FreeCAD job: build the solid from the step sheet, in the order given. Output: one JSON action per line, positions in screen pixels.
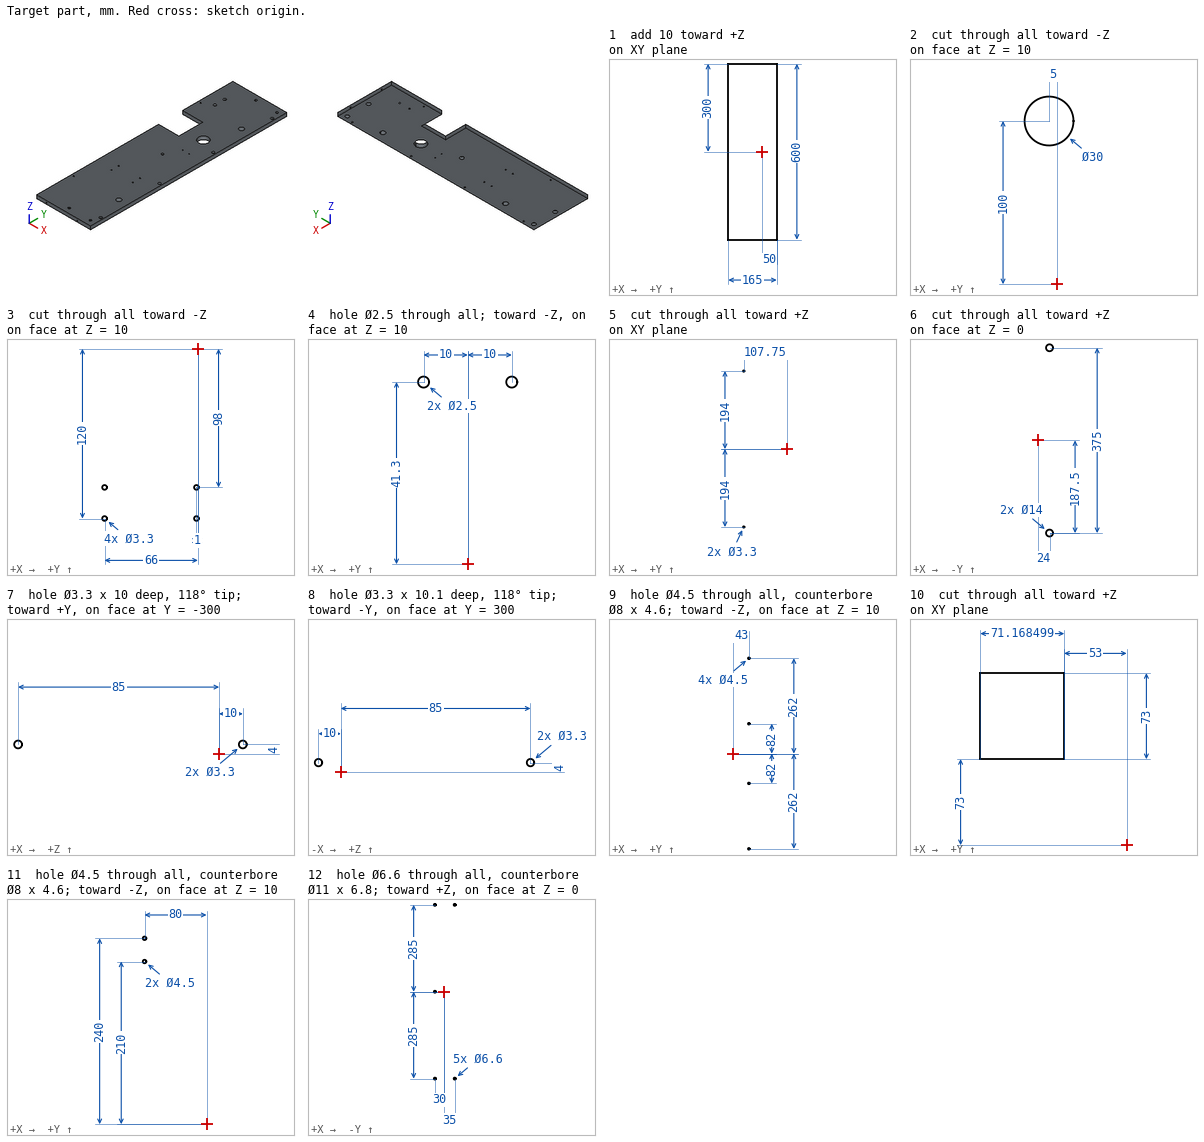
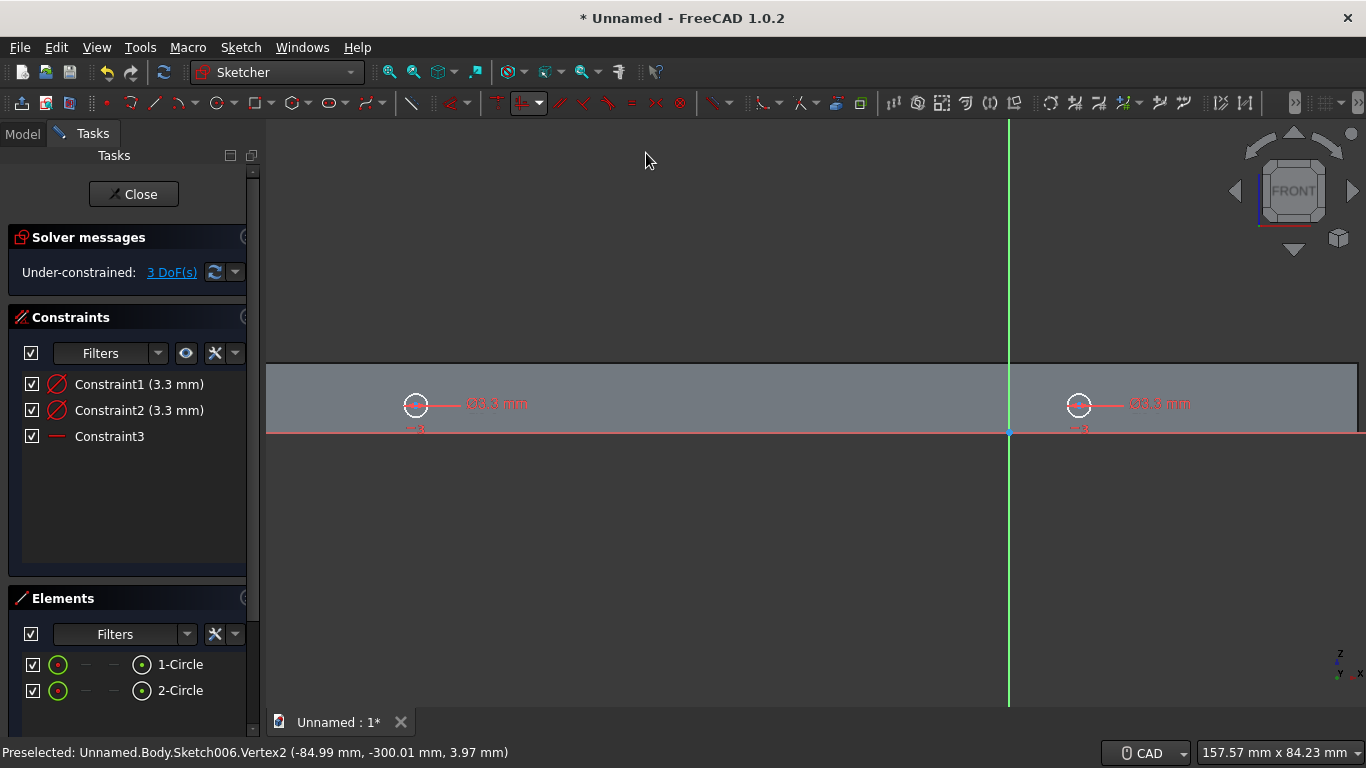
{"action": "left_click", "coordinate": [450, 104]}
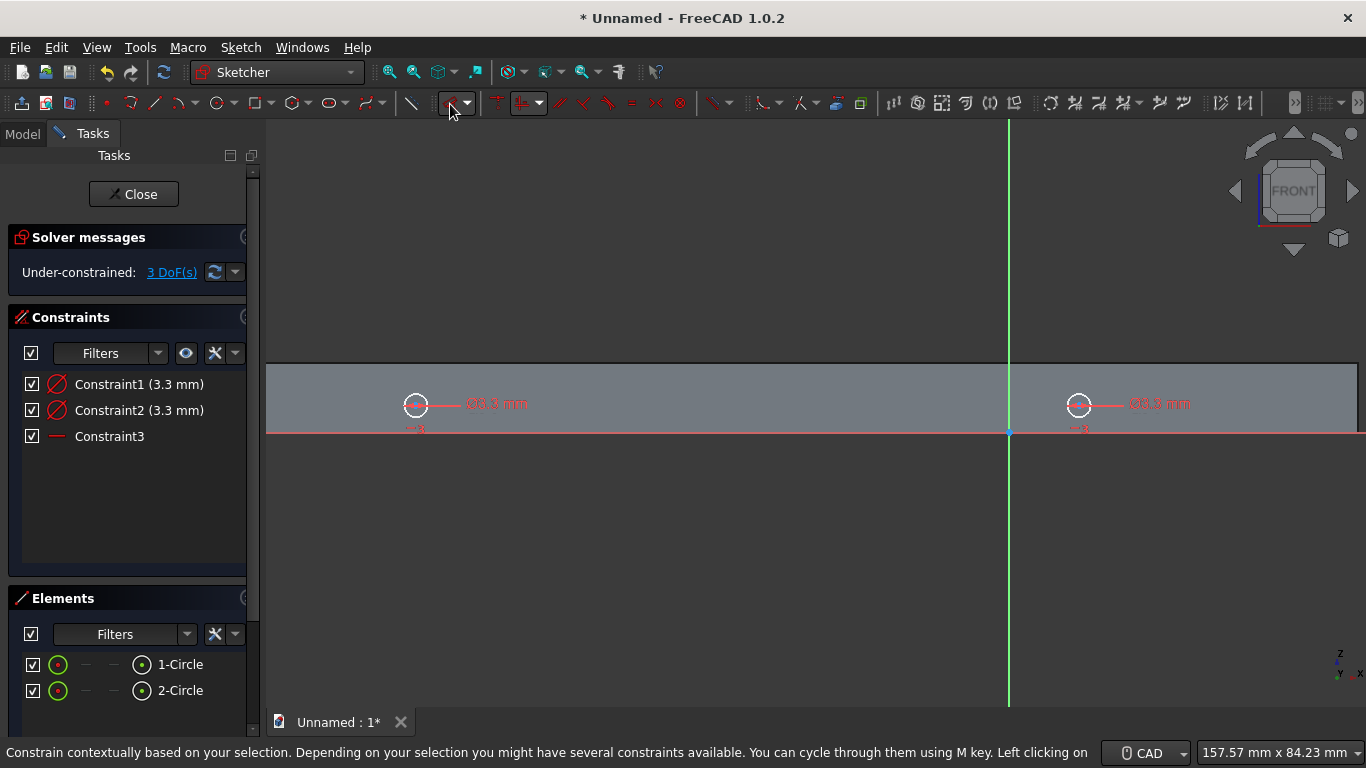
{"action": "scroll", "coordinate": [1079, 406], "scroll_direction": "up", "scroll_amount": 2}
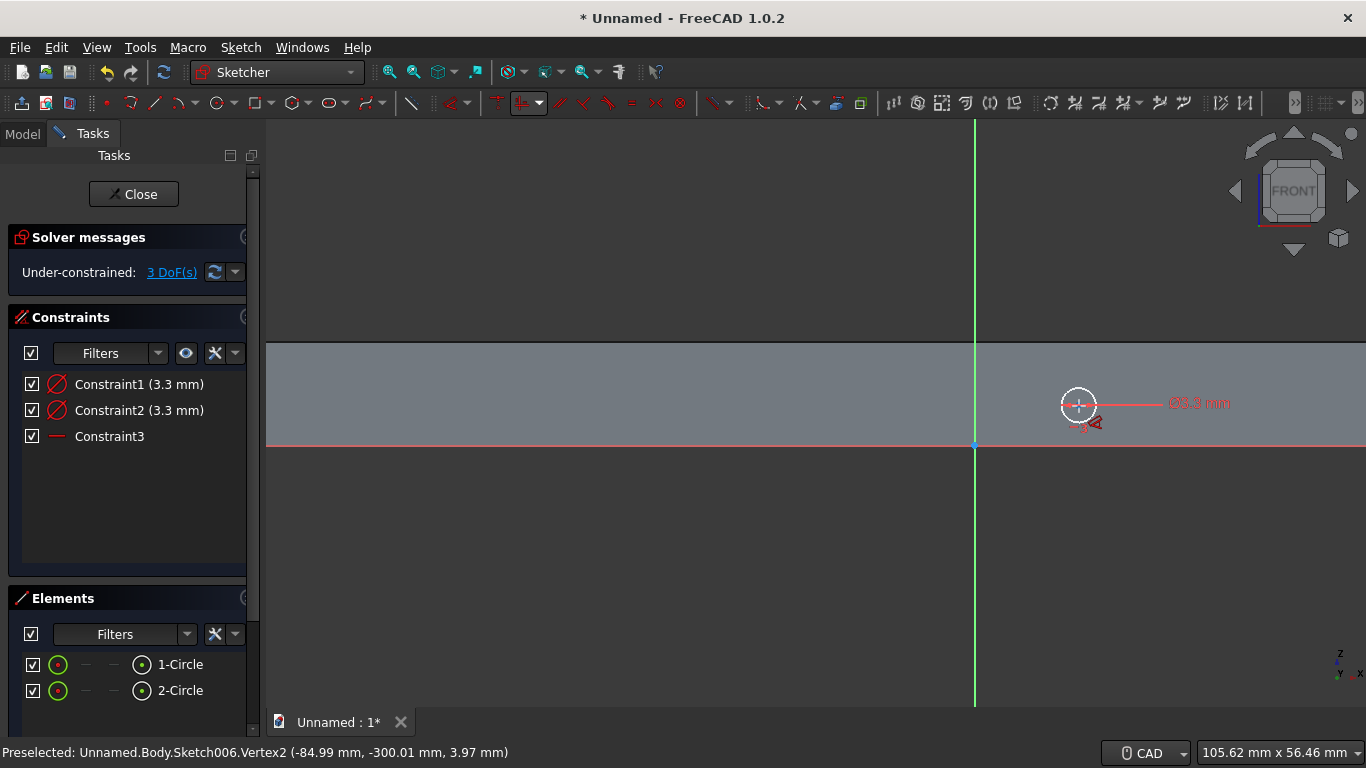
{"action": "left_click", "coordinate": [1079, 405]}
{"action": "left_click", "coordinate": [1113, 426]}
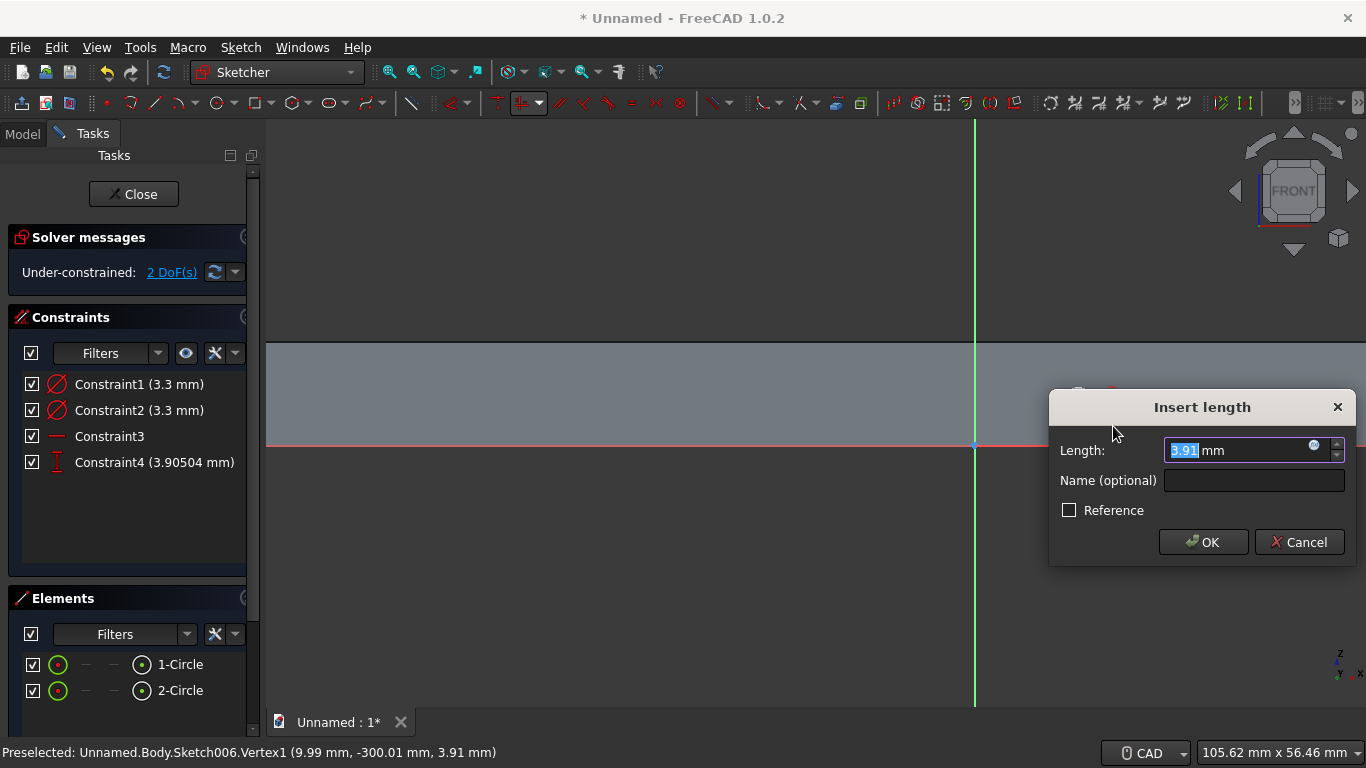
{"action": "type", "text": "4"}
{"action": "key", "text": "Return"}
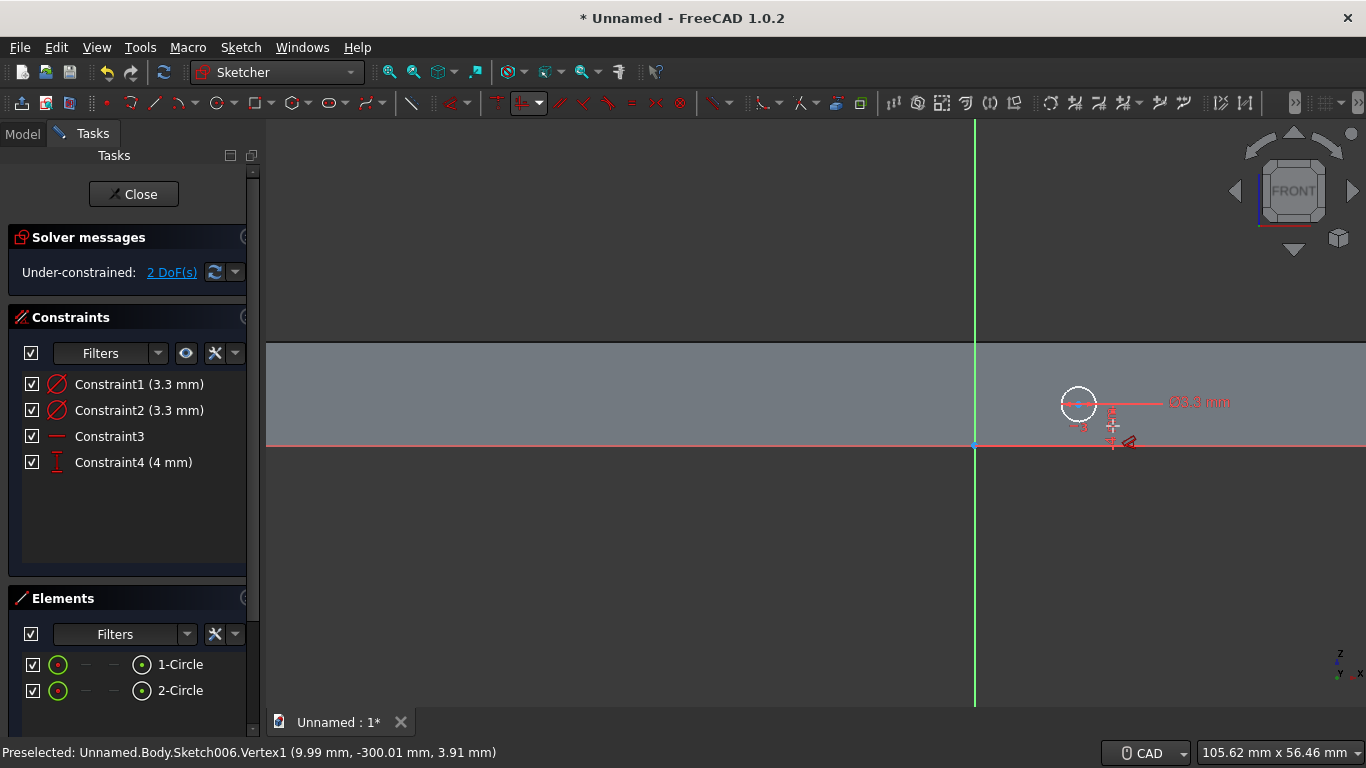
{"action": "left_click", "coordinate": [1079, 404]}
{"action": "left_click", "coordinate": [1027, 480]}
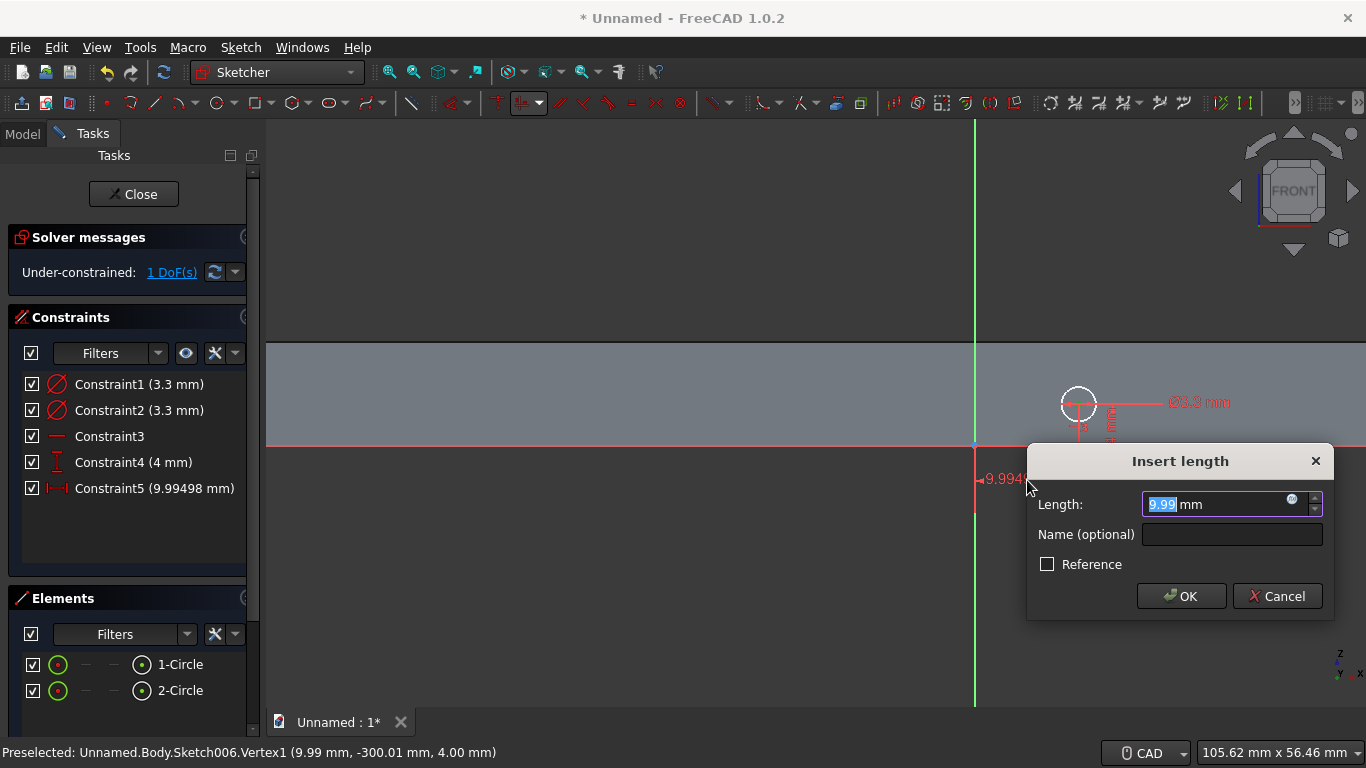
{"action": "type", "text": "10"}
{"action": "key", "text": "Return"}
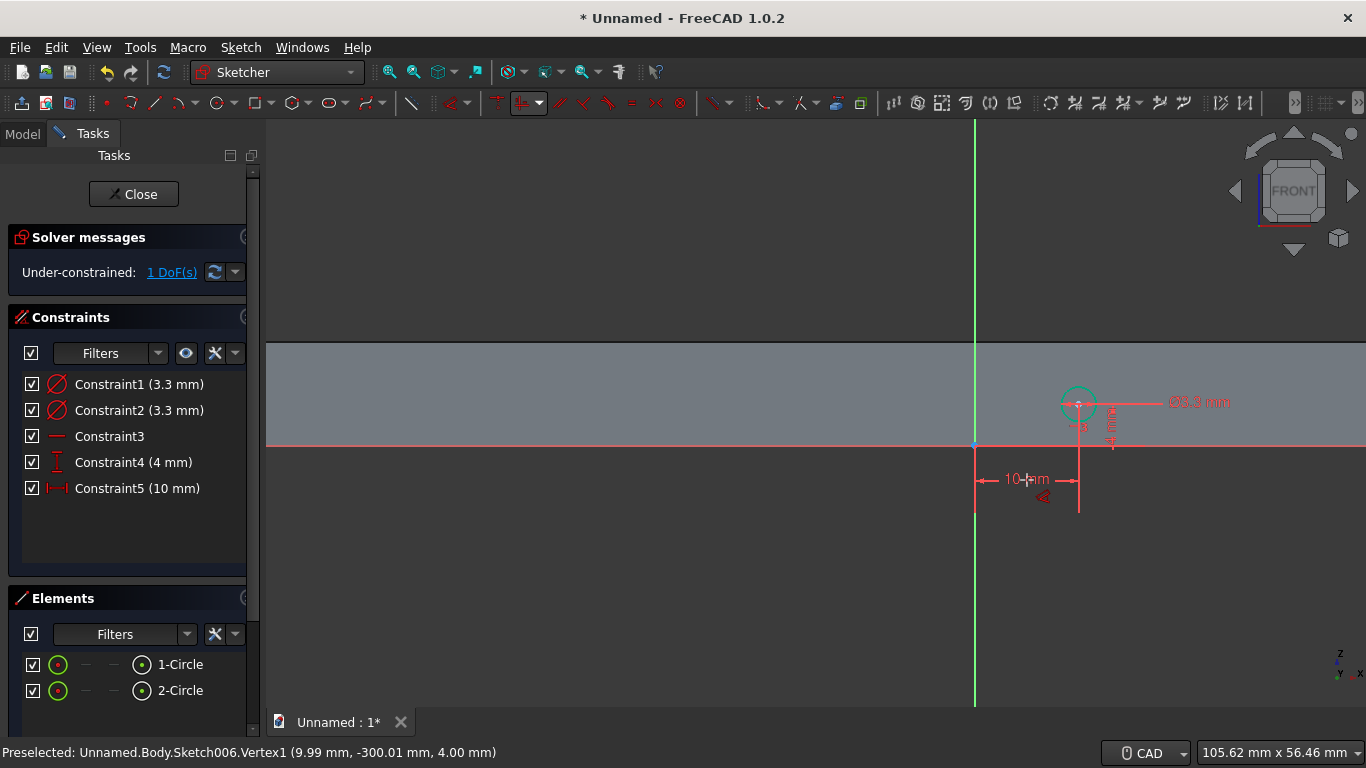
{"action": "scroll", "coordinate": [1080, 406], "scroll_direction": "down", "scroll_amount": 2}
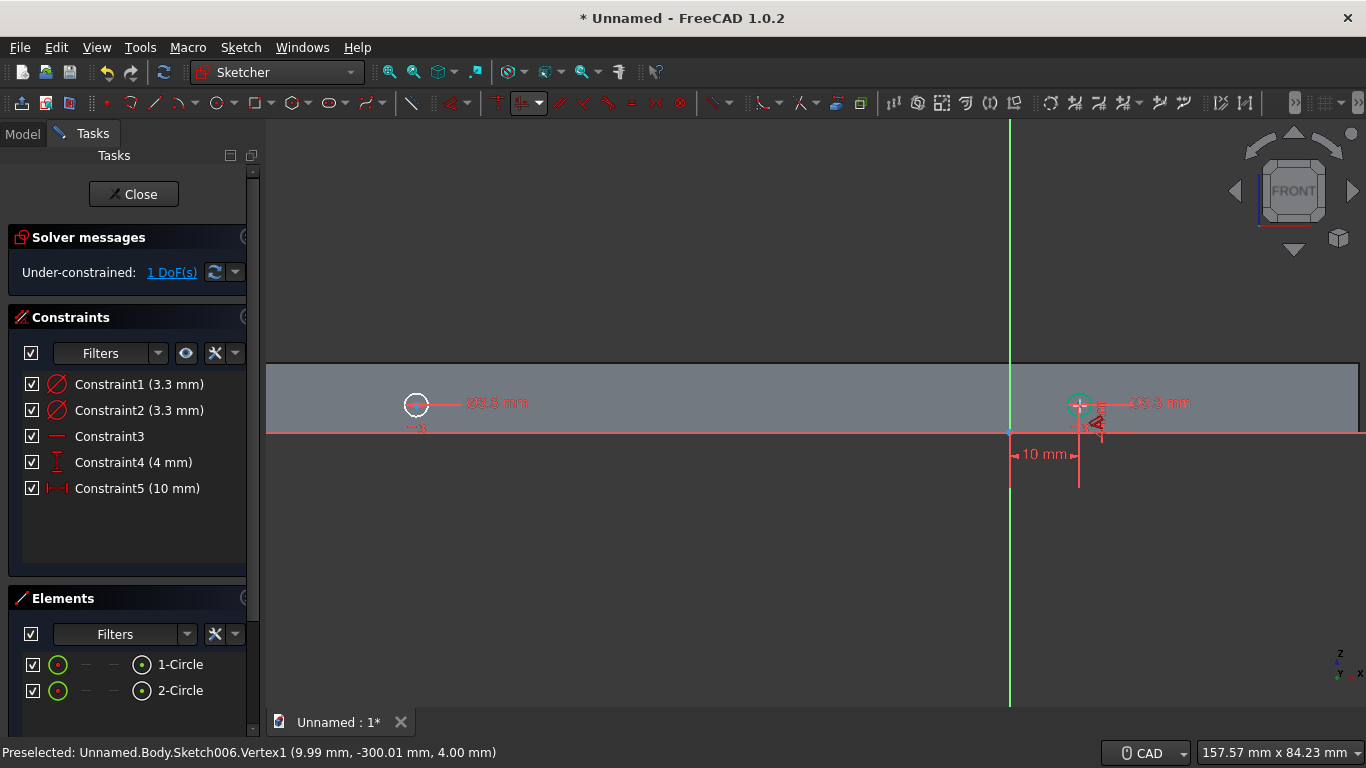
{"action": "left_click", "coordinate": [416, 405]}
{"action": "left_click", "coordinate": [713, 467]}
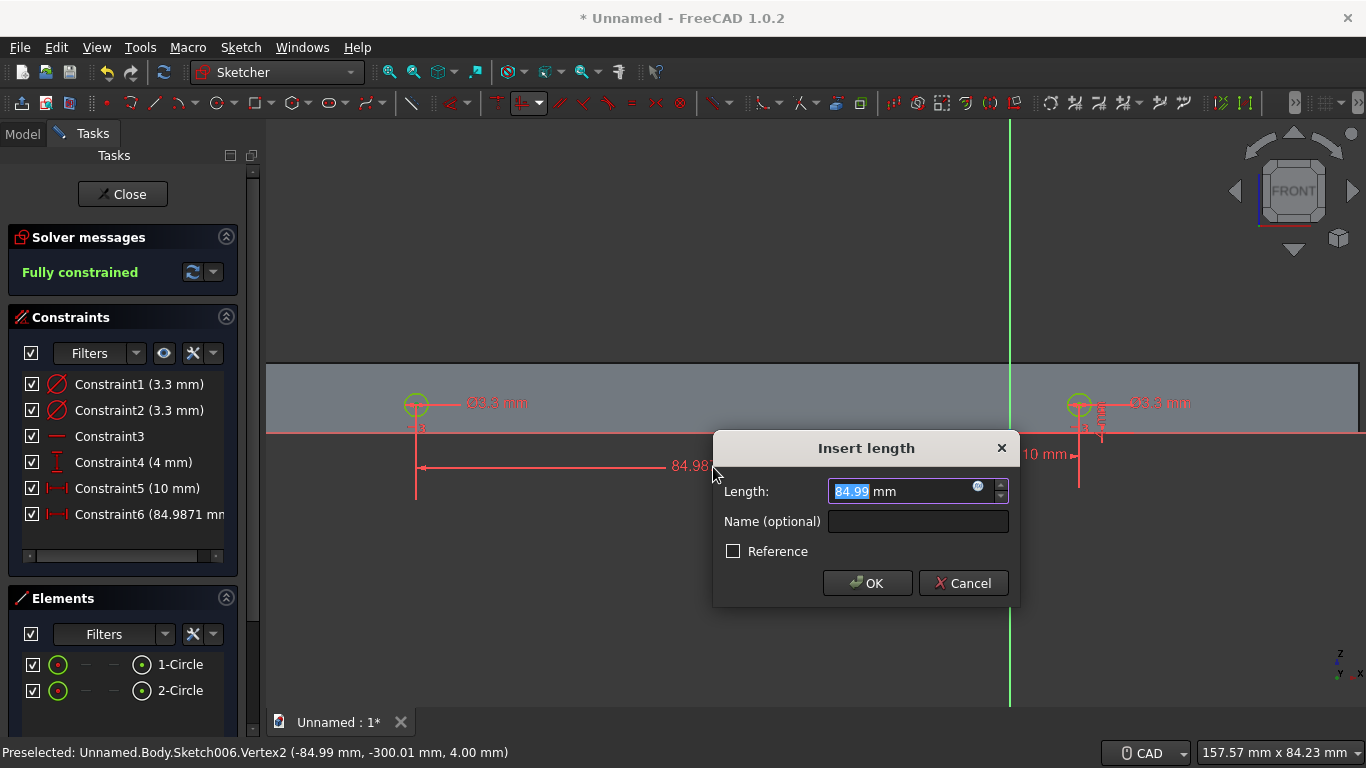
{"action": "type", "text": "85"}
{"action": "key", "text": "Return"}
{"action": "key", "text": "Escape"}